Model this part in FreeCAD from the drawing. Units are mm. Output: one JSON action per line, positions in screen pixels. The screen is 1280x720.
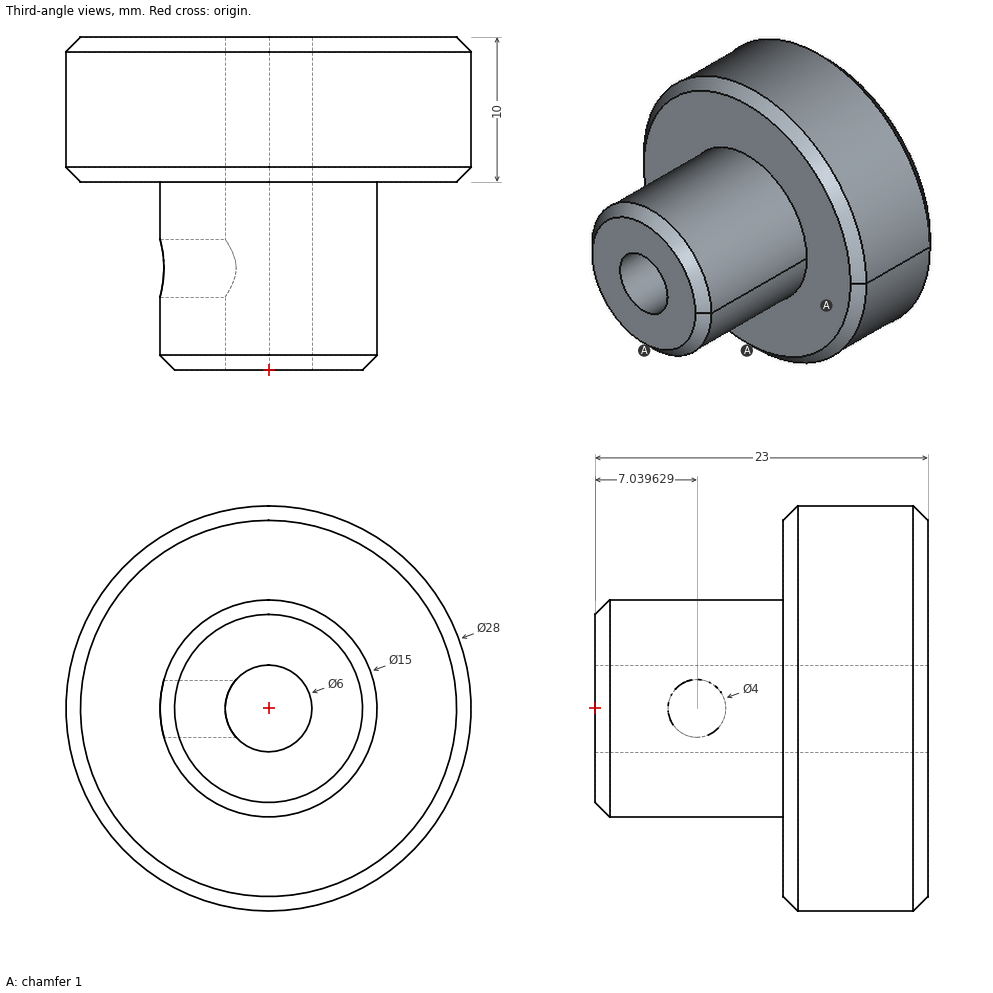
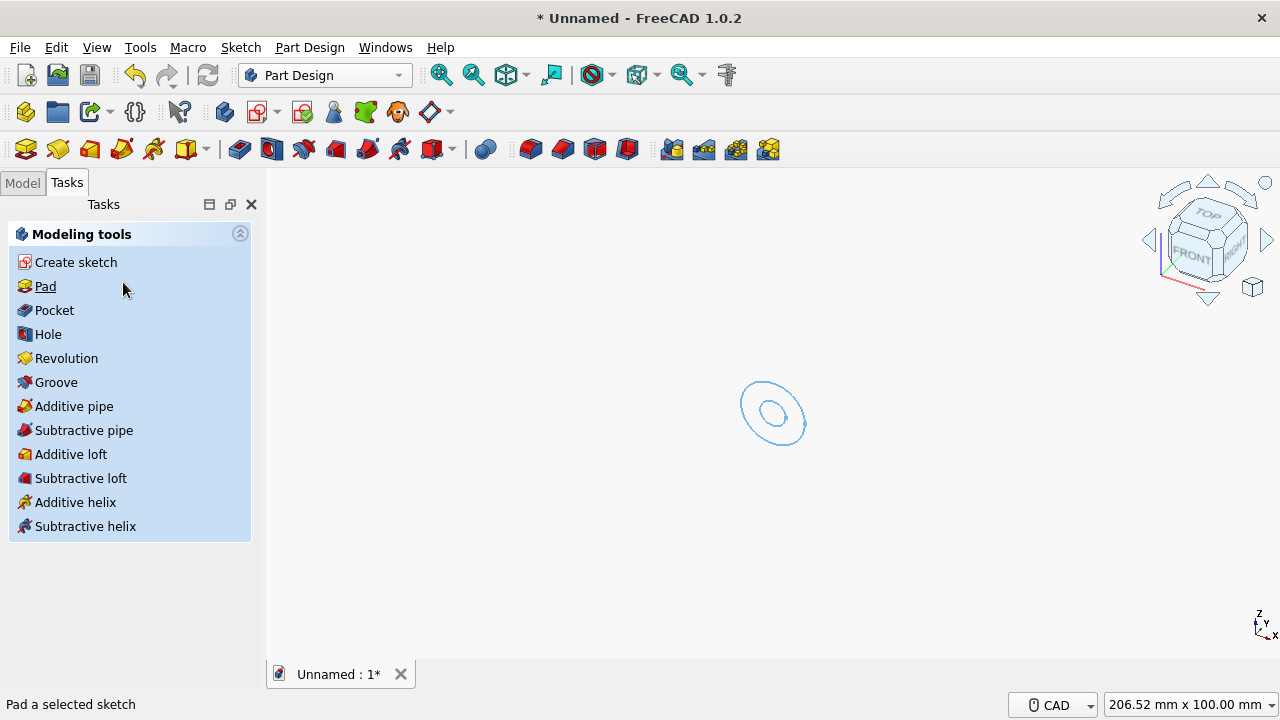
{"action": "left_click", "coordinate": [26, 150]}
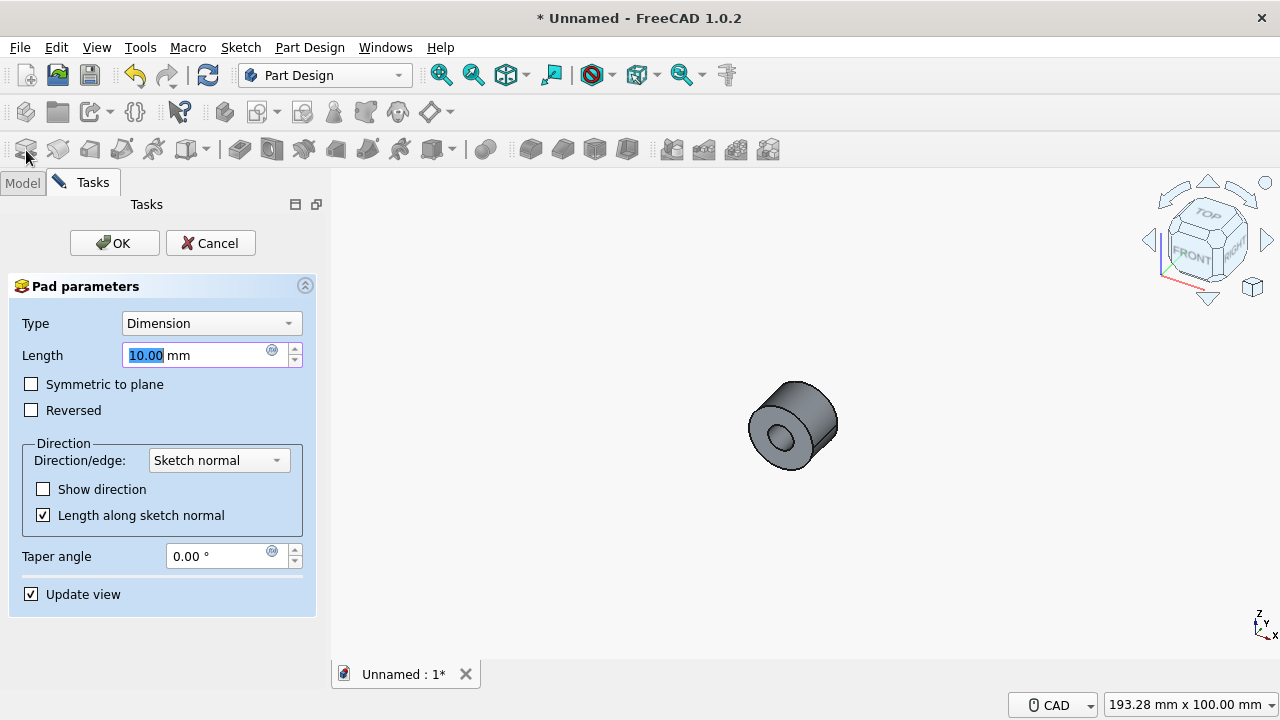
{"action": "type", "text": "23"}
{"action": "key", "text": "Tab"}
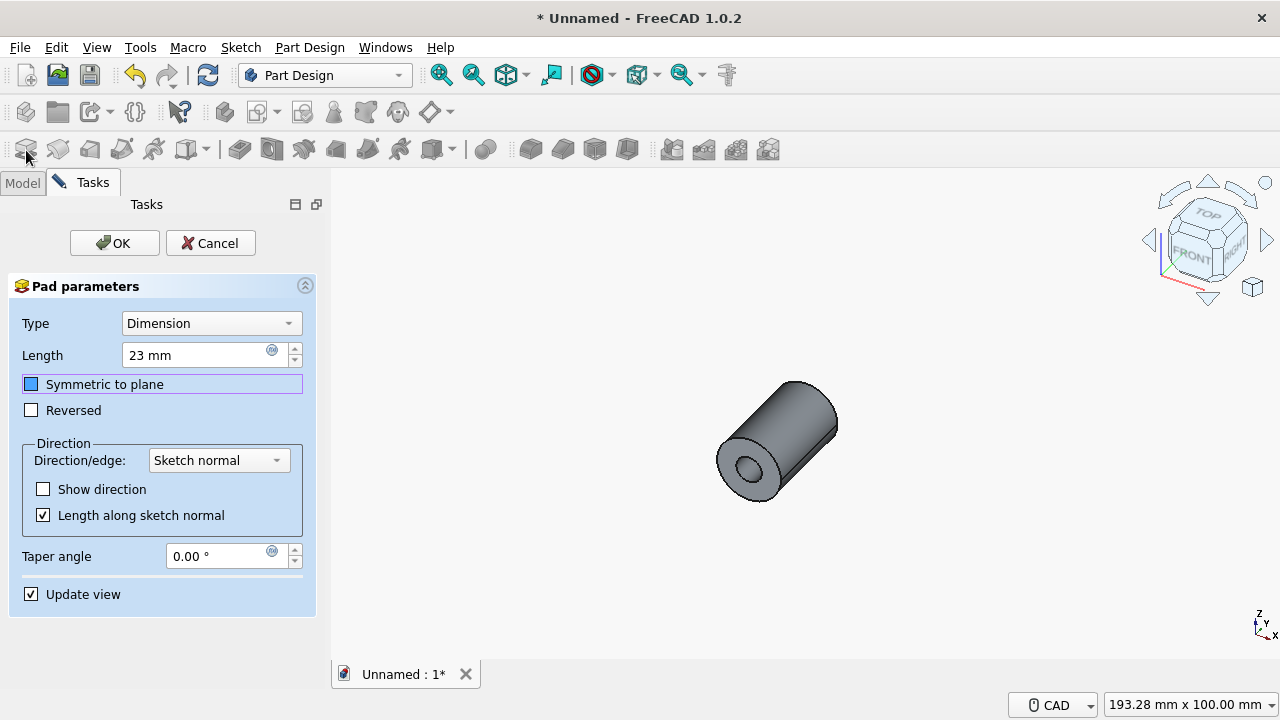
{"action": "left_click", "coordinate": [30, 410]}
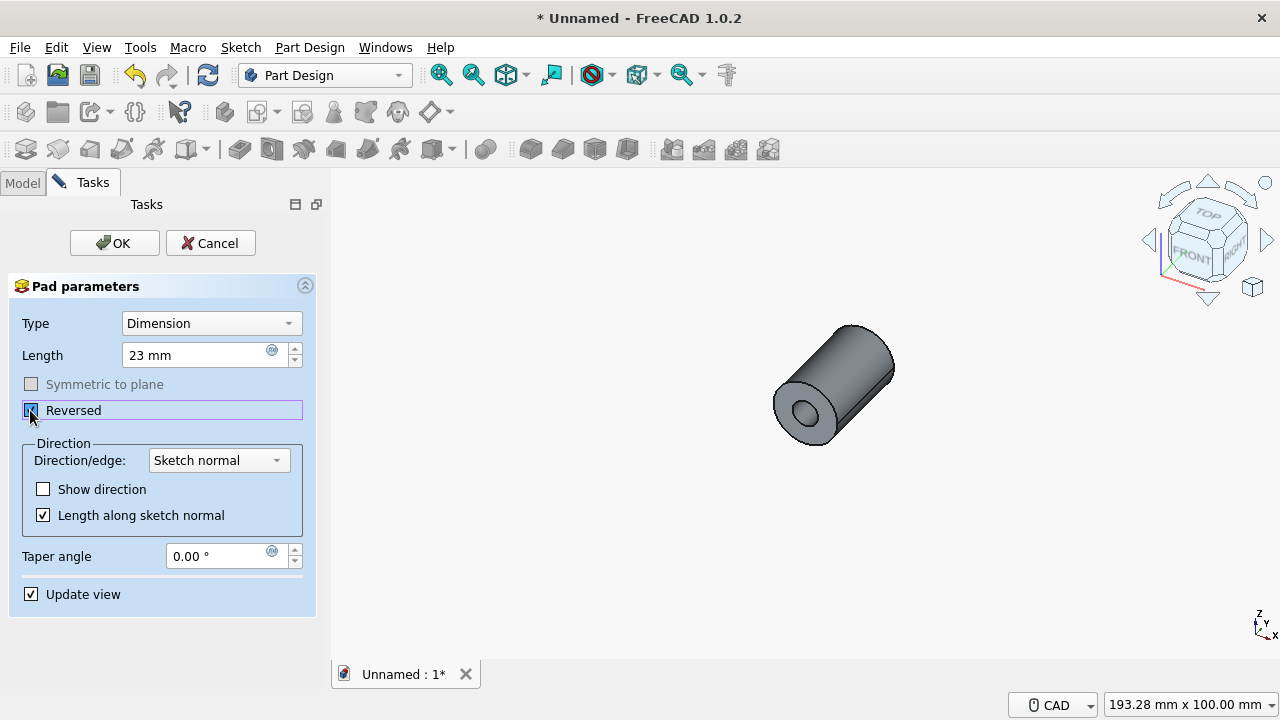
{"action": "left_click", "coordinate": [115, 243]}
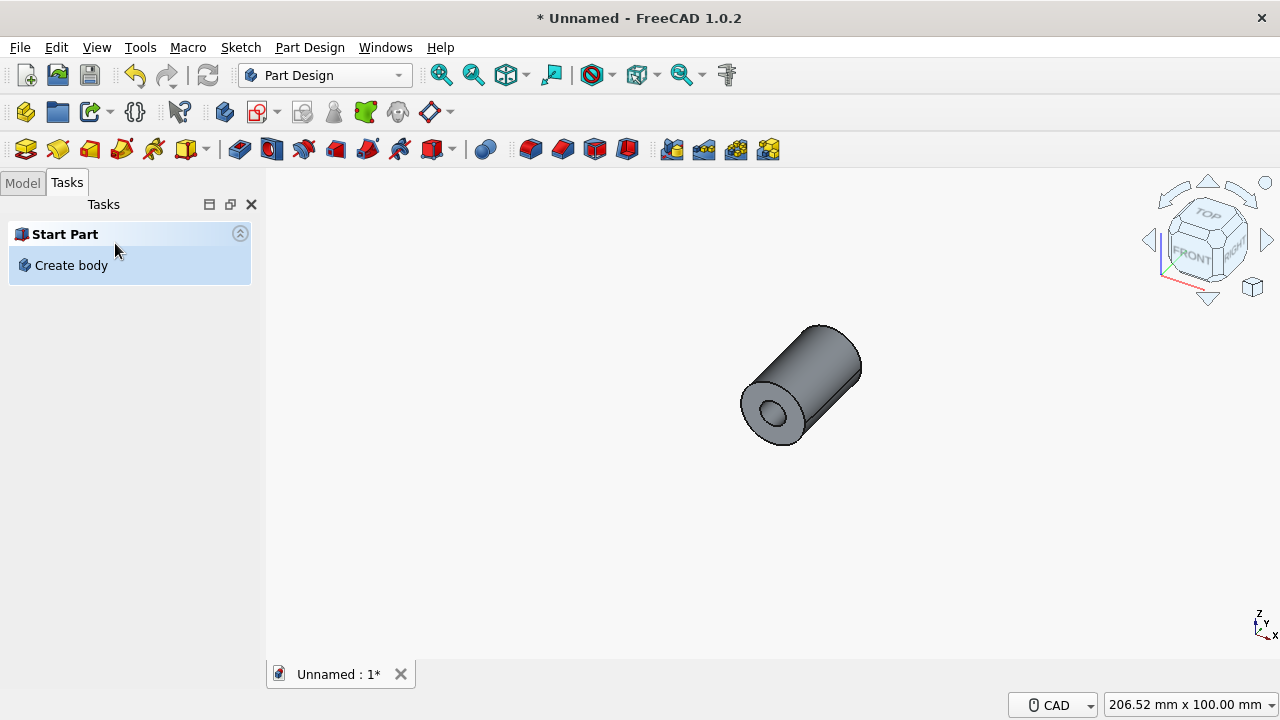
{"action": "left_click", "coordinate": [442, 76]}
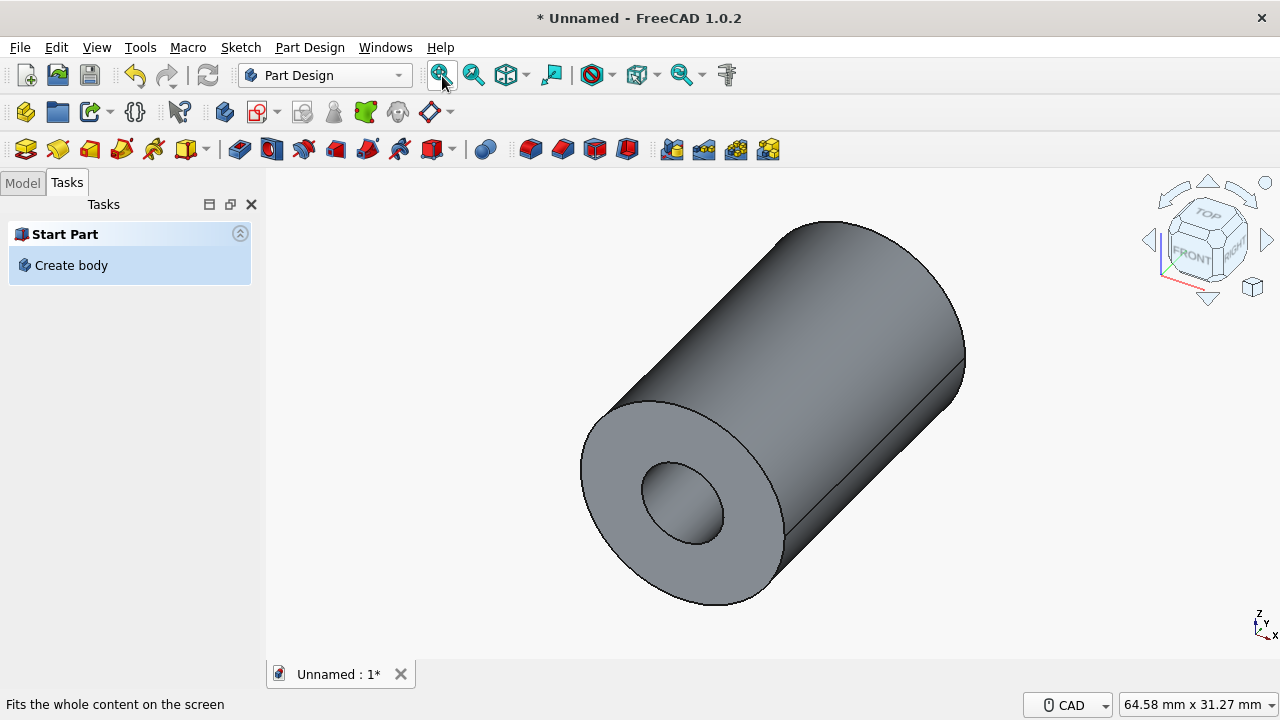
{"action": "left_click", "coordinate": [23, 182]}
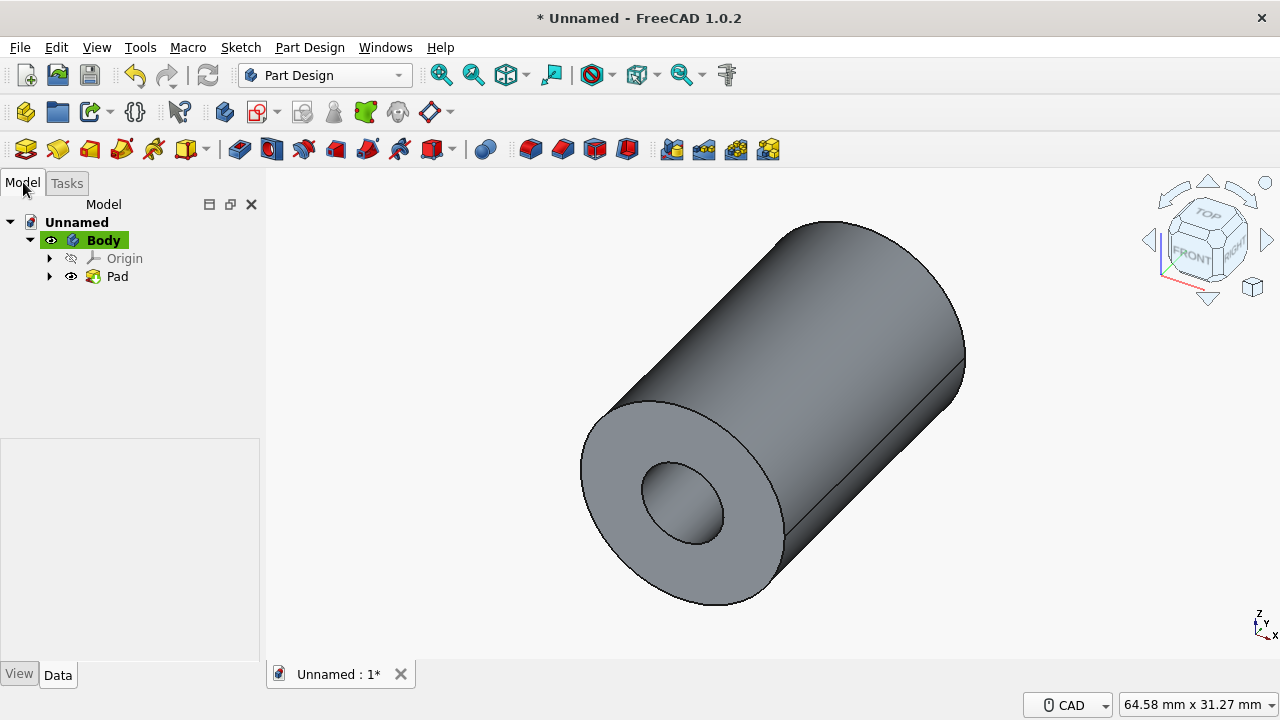
{"action": "left_click", "coordinate": [50, 258]}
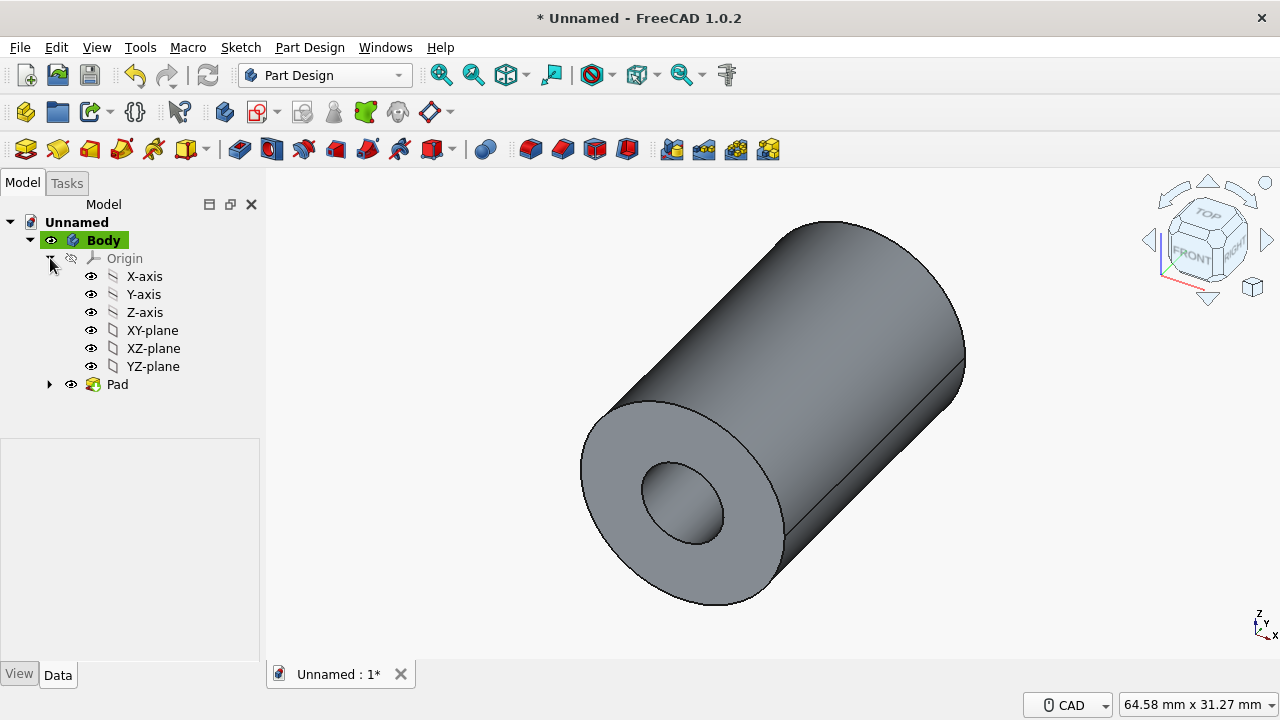
{"action": "left_click", "coordinate": [136, 348]}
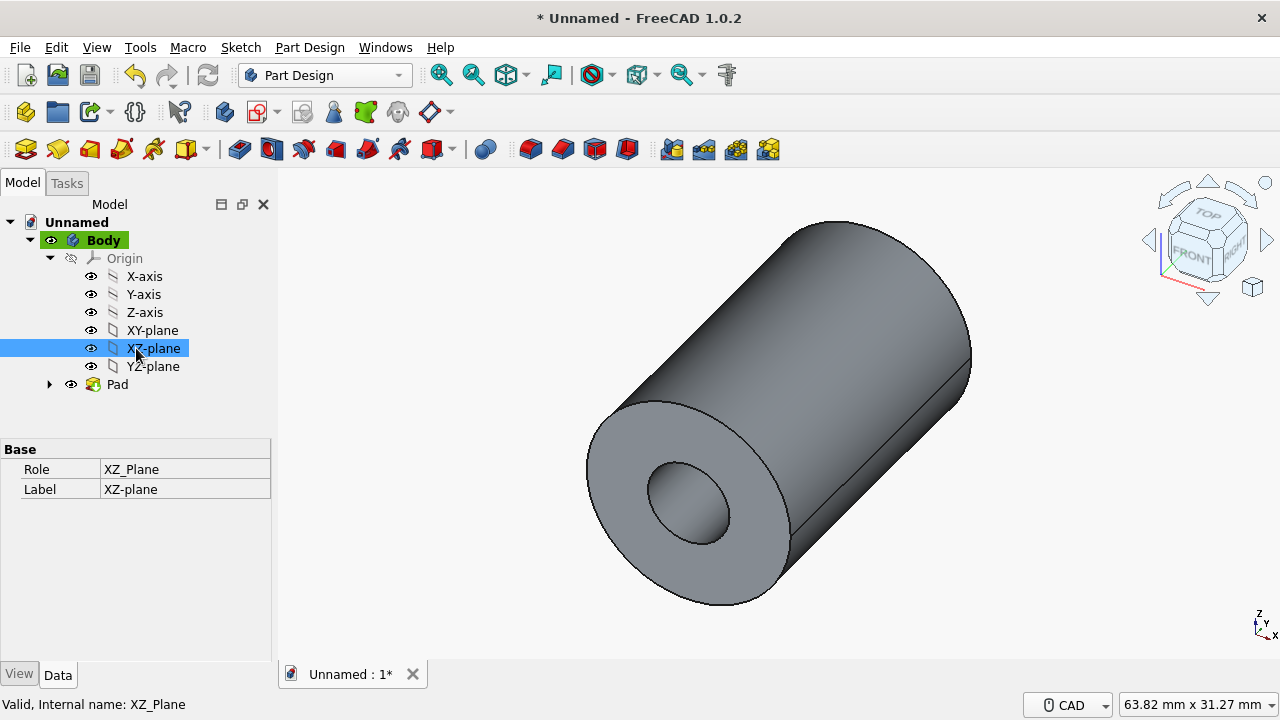
{"action": "left_click", "coordinate": [430, 112]}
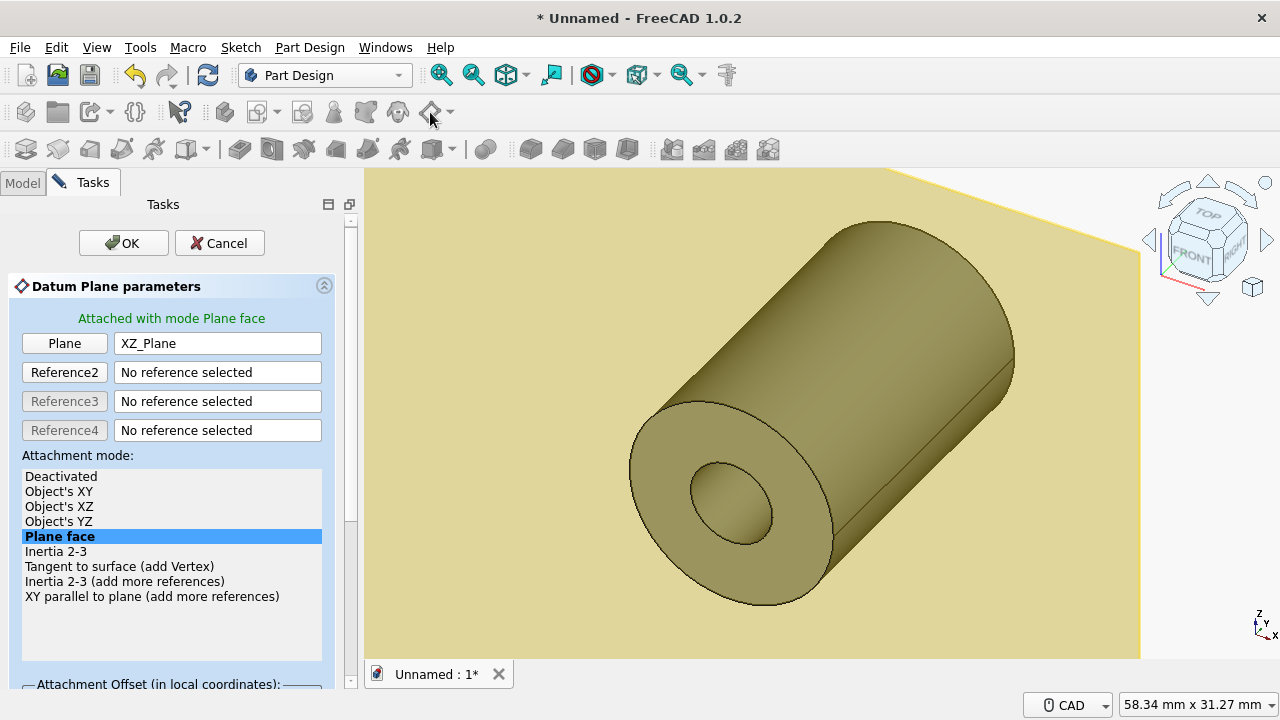
{"action": "scroll", "coordinate": [351, 451], "scroll_direction": "down", "scroll_amount": 3}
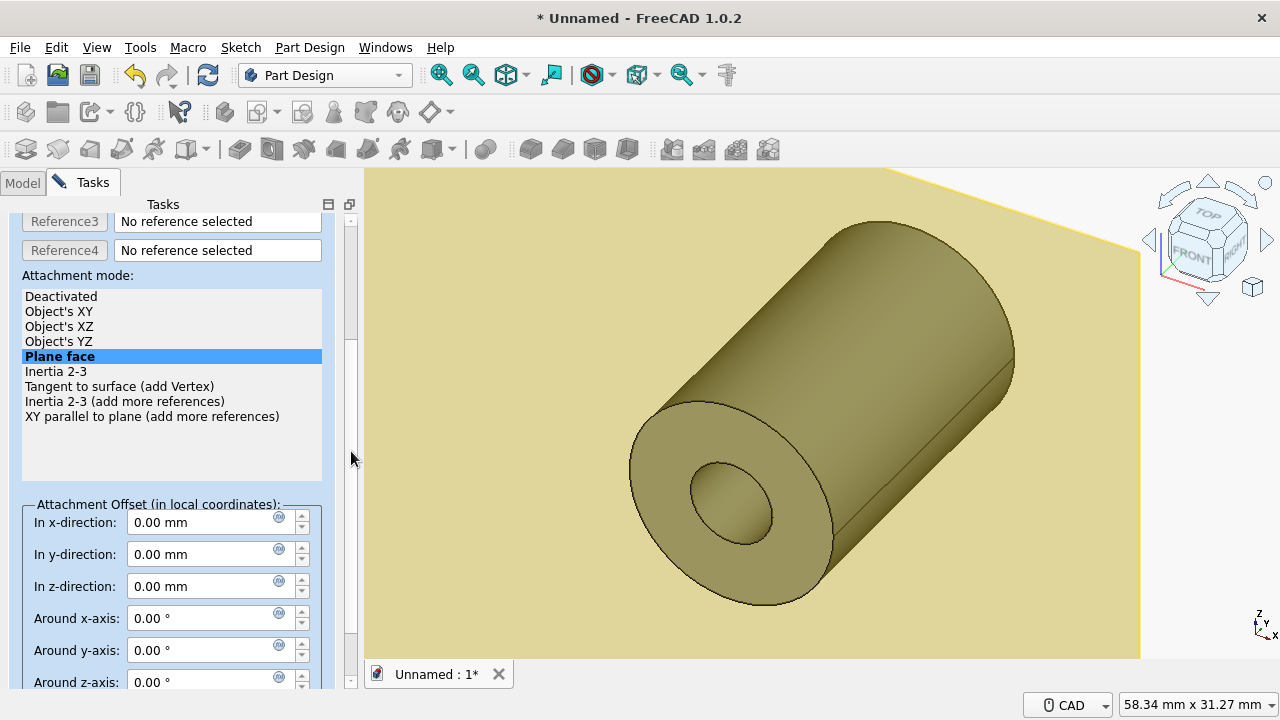
{"action": "triple_click", "coordinate": [210, 586]}